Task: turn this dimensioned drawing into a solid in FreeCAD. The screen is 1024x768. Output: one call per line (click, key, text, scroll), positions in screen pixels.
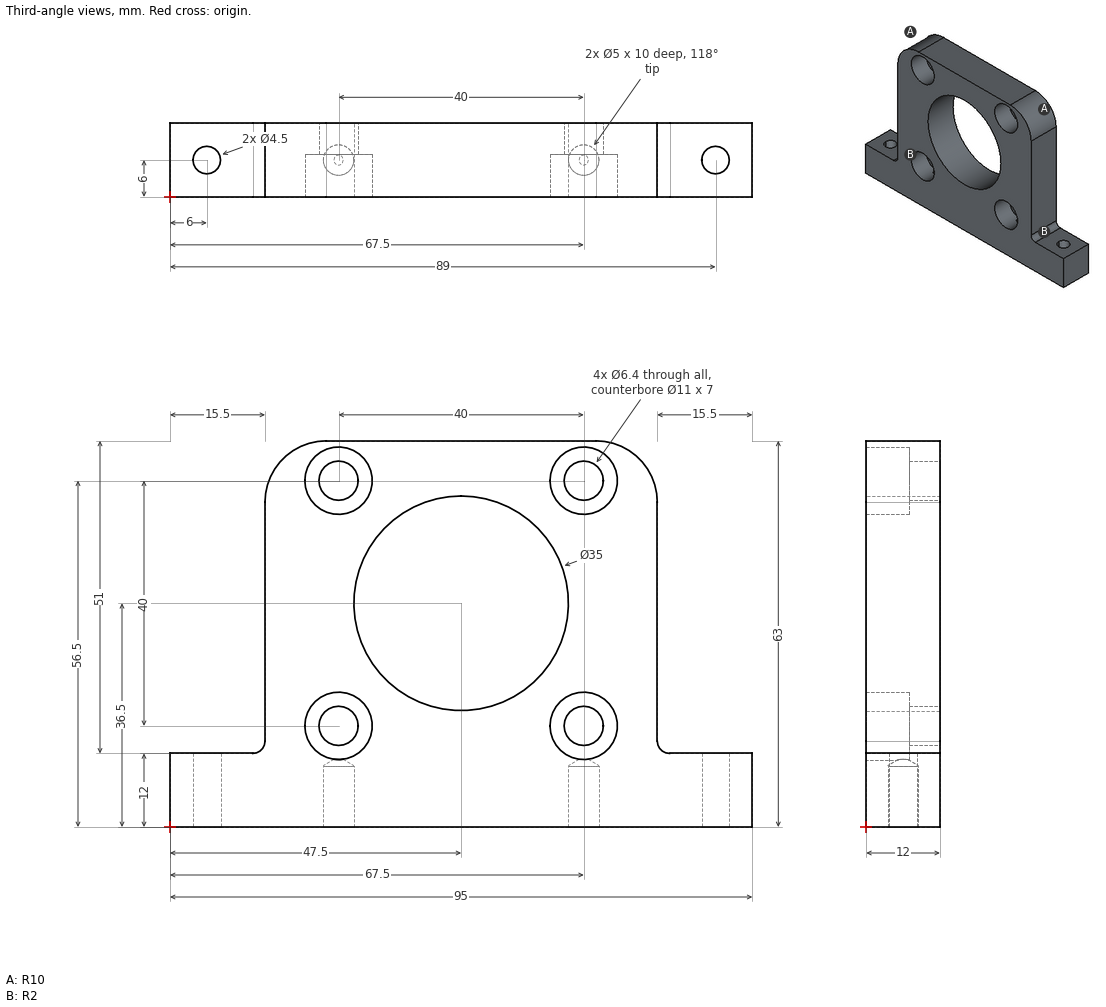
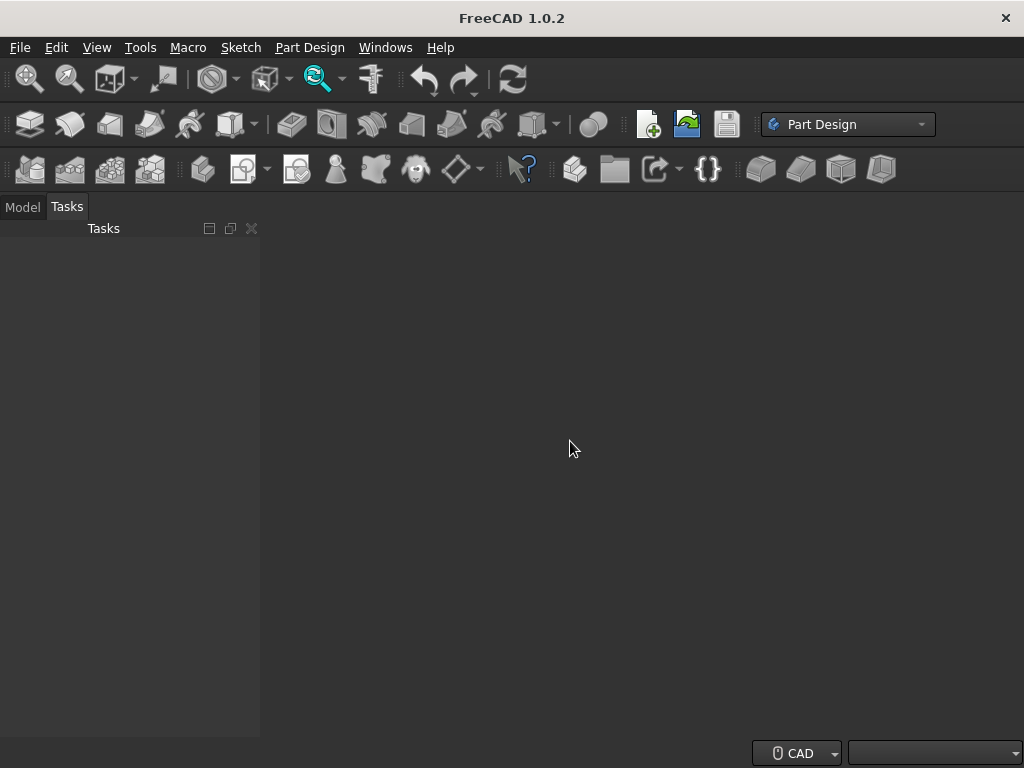
click(648, 124)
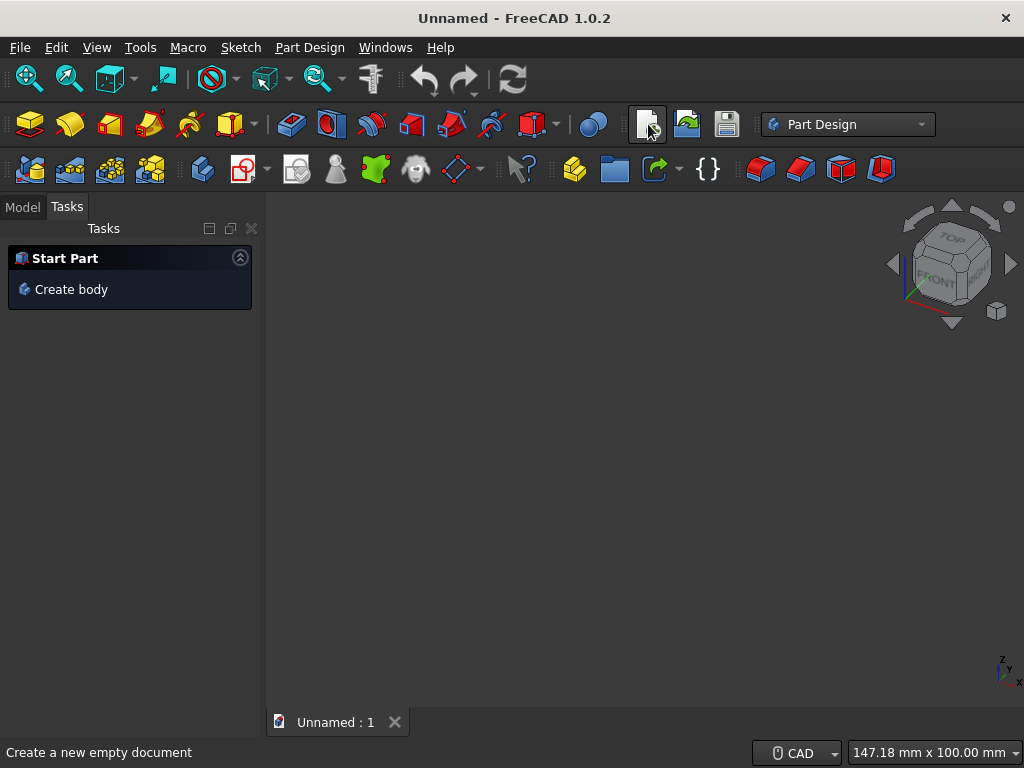
click(244, 170)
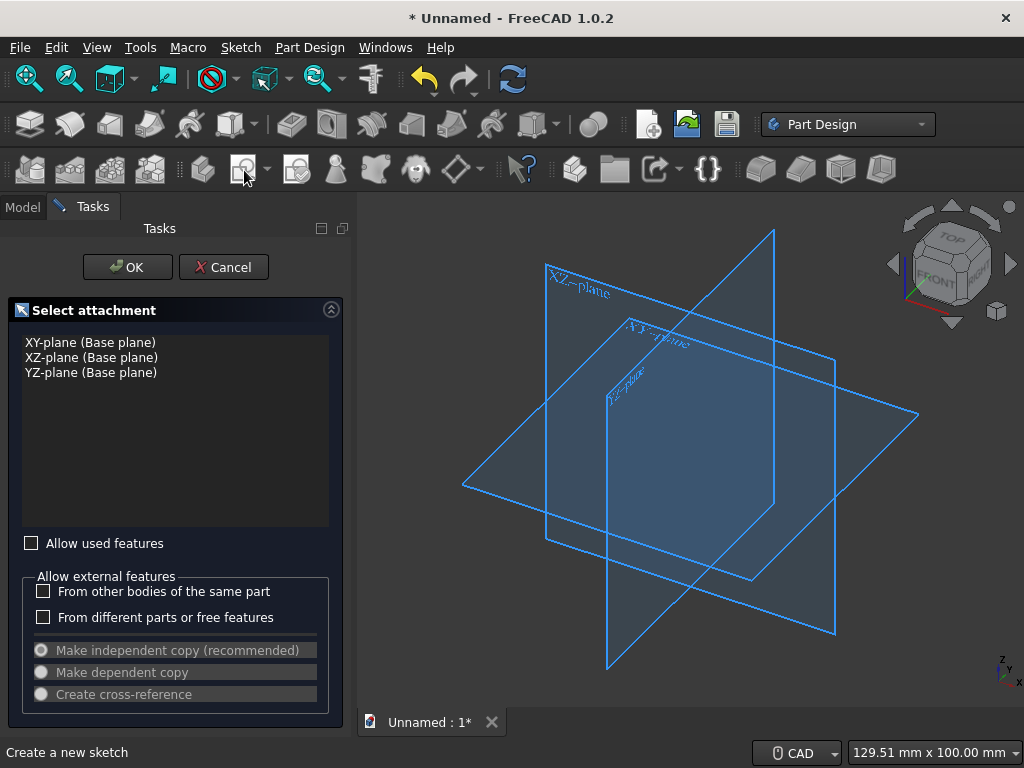
click(82, 358)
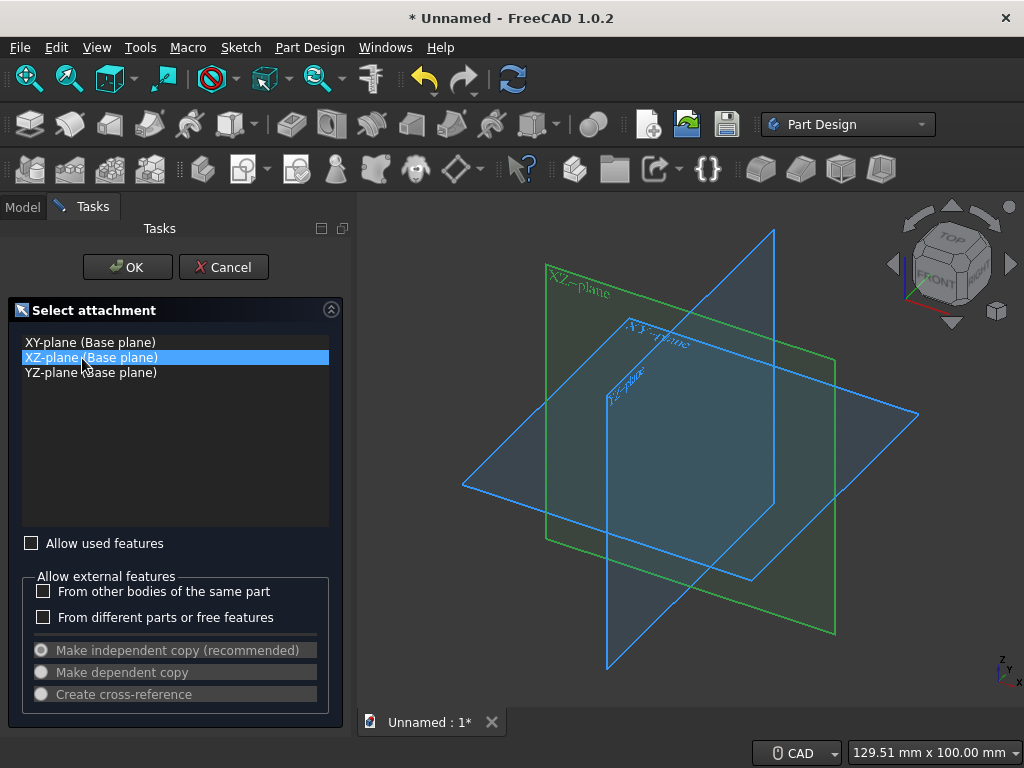
click(128, 267)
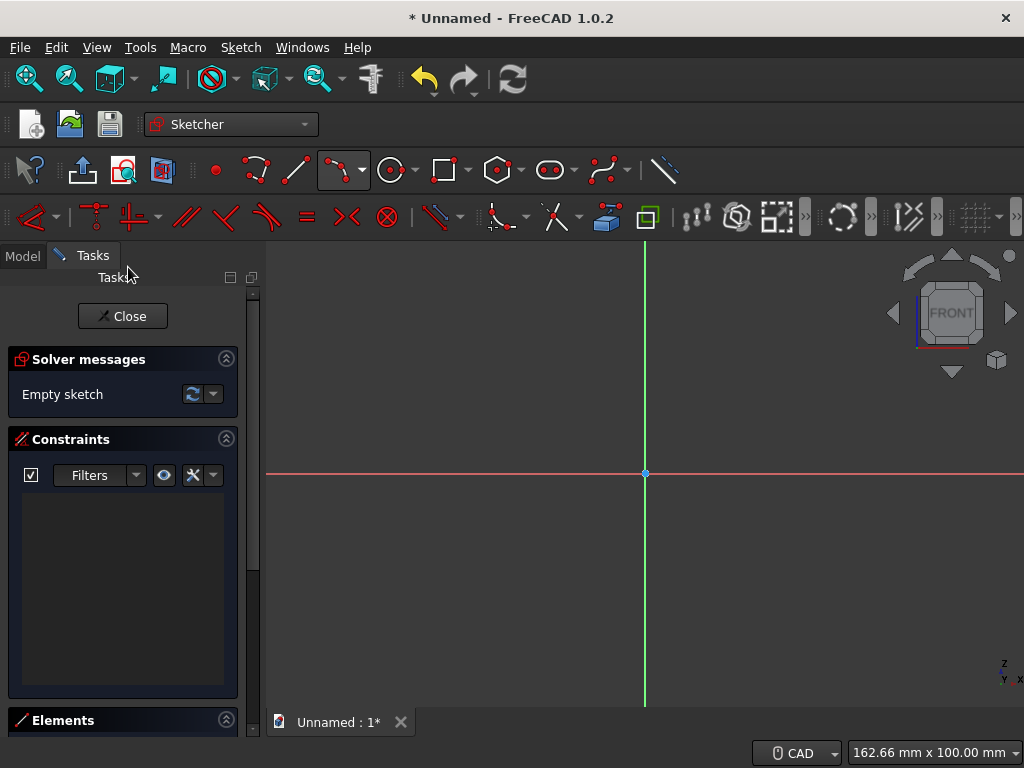
scroll(294, 679, down, 2)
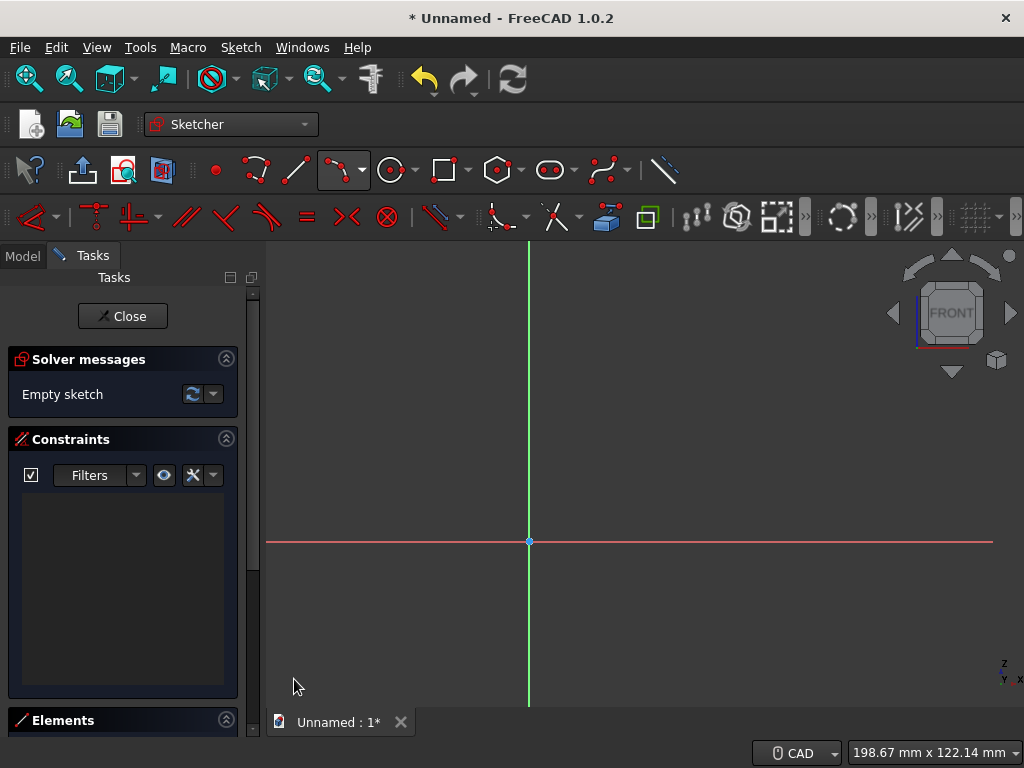
click(444, 170)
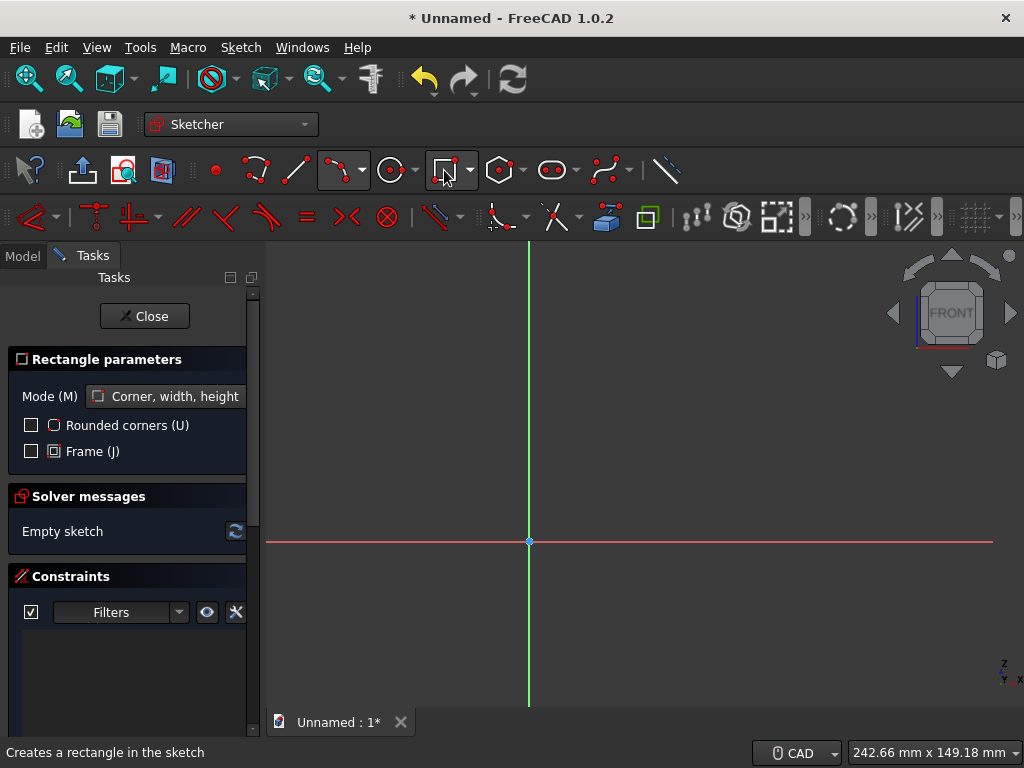
click(529, 542)
click(826, 345)
key(Escape)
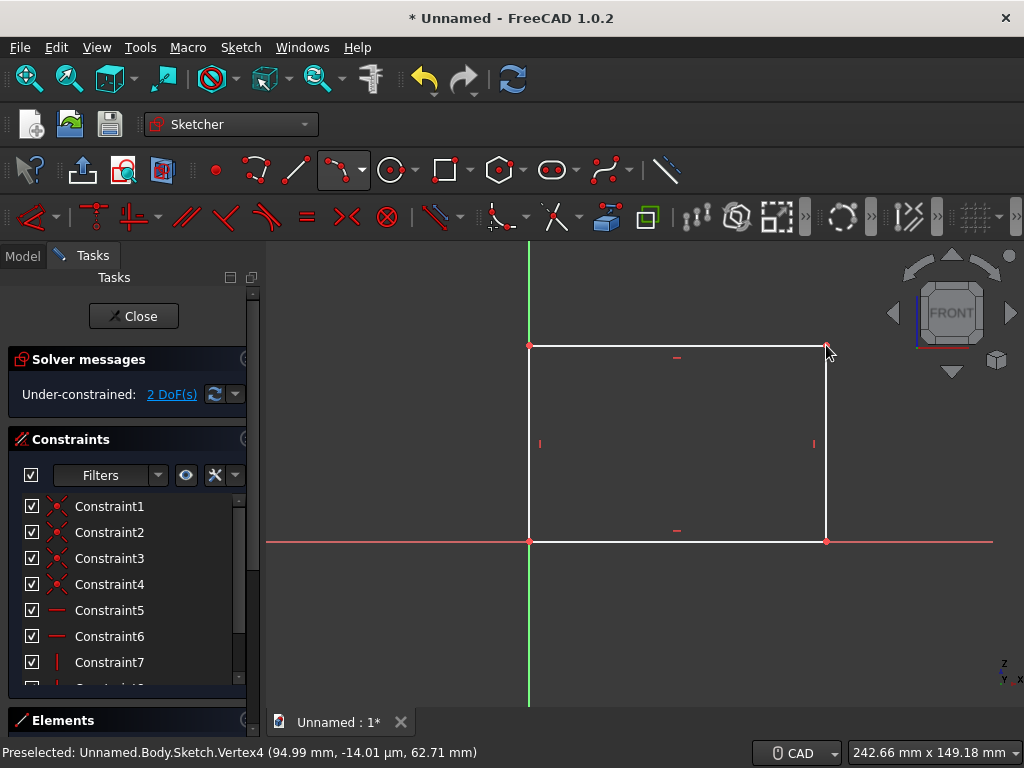
key(d)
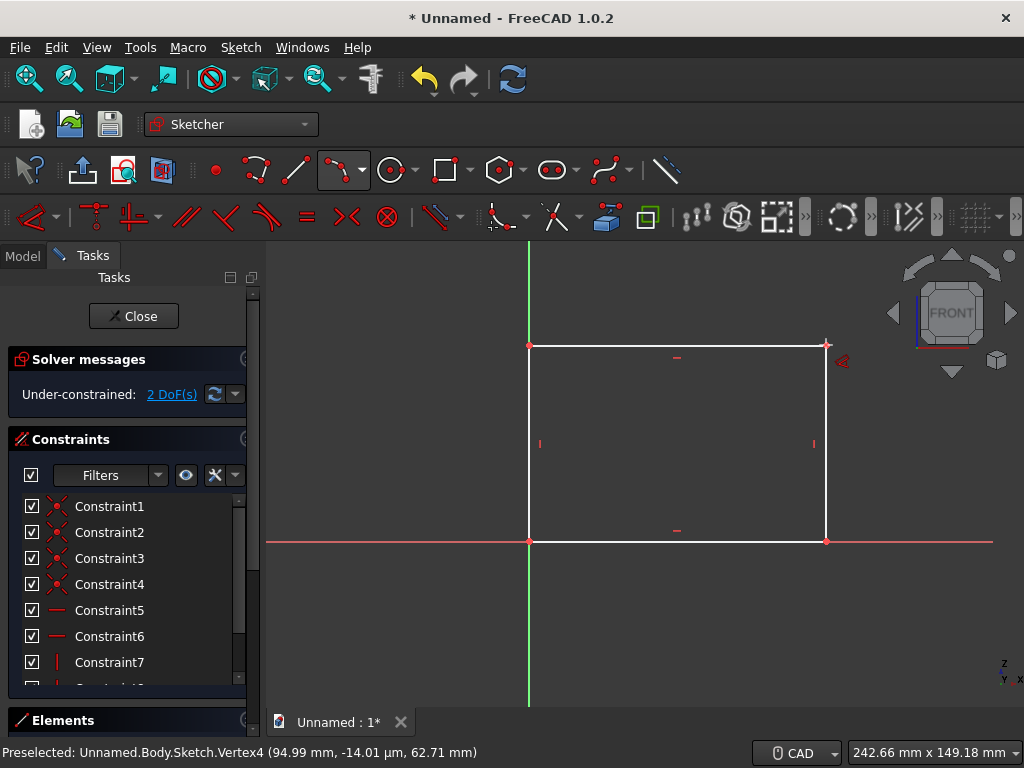
click(618, 542)
click(678, 576)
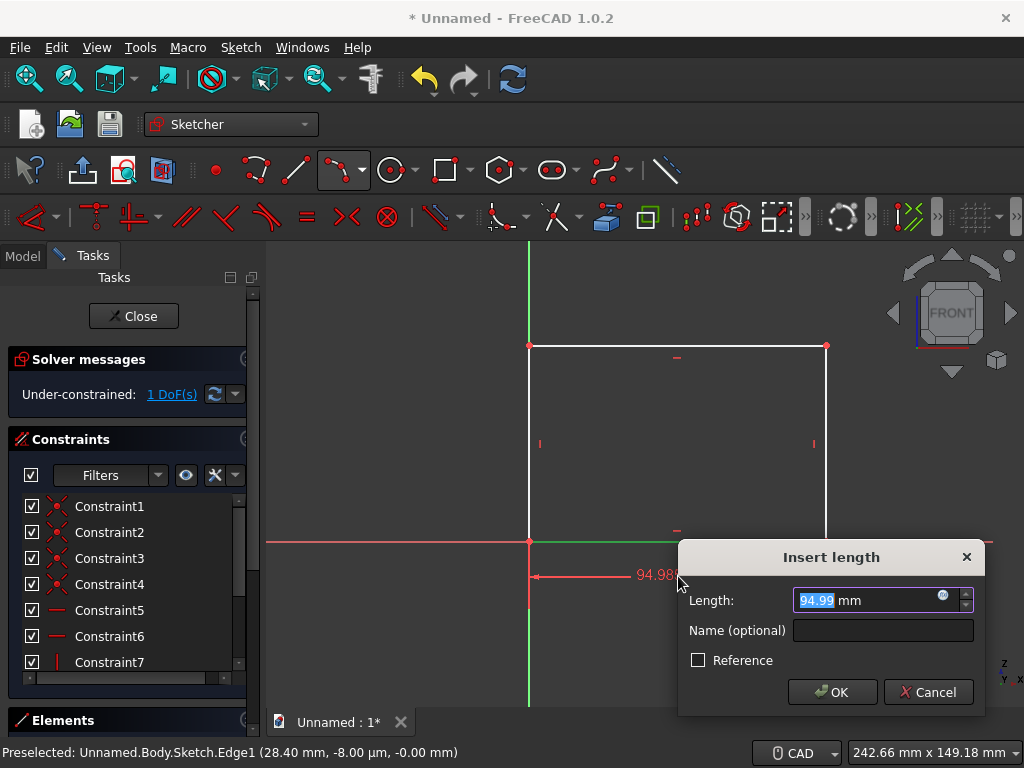
text(95)
key(Return)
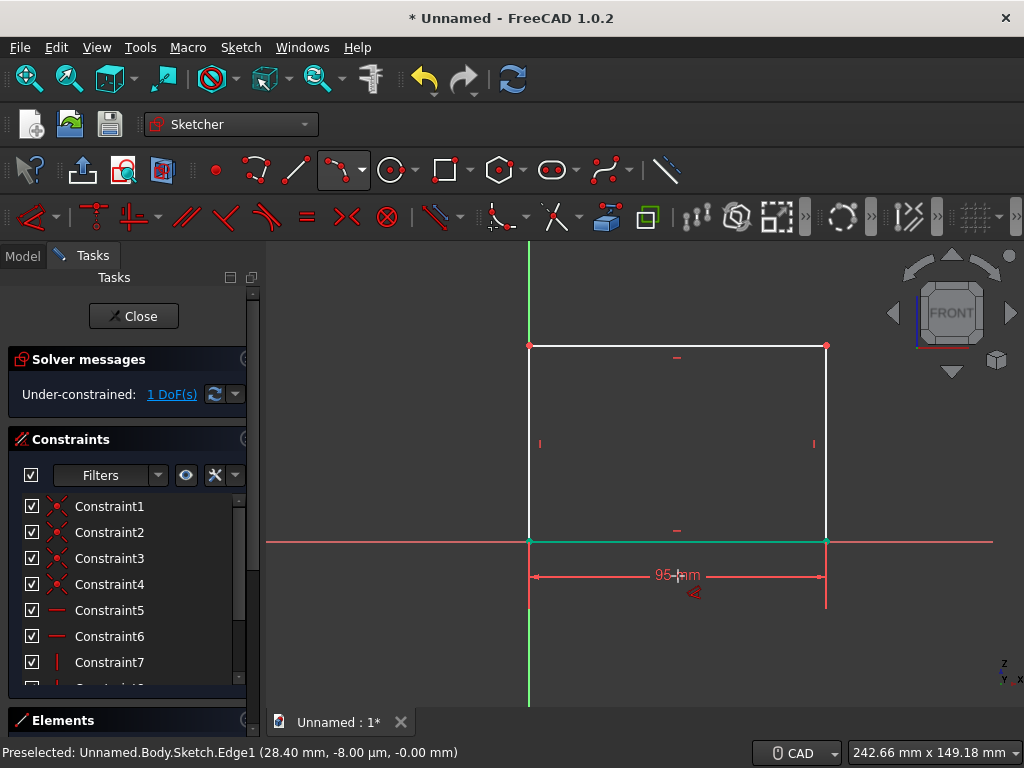
click(826, 483)
click(792, 444)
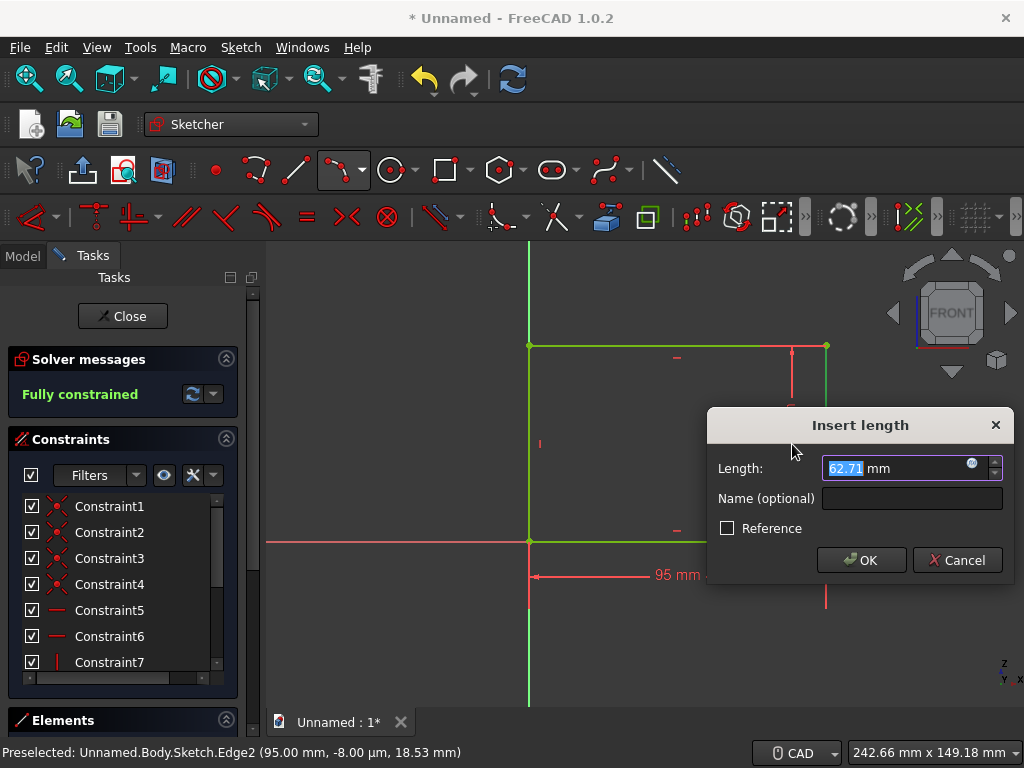
text(63)
key(Return)
key(Escape)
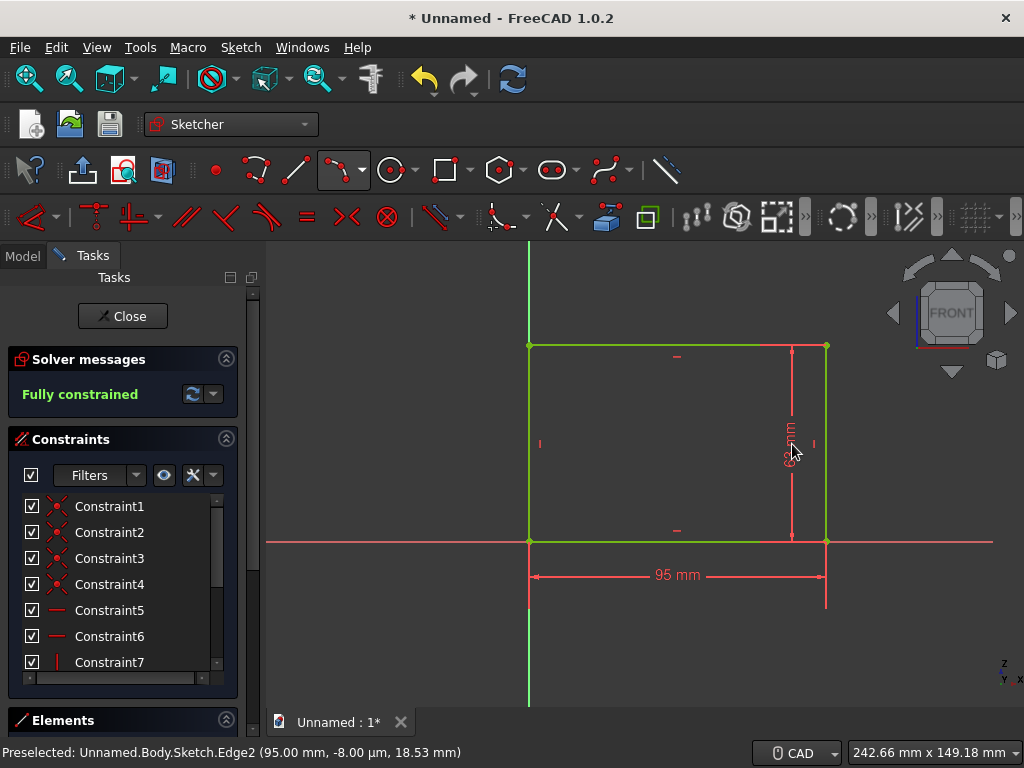
click(123, 316)